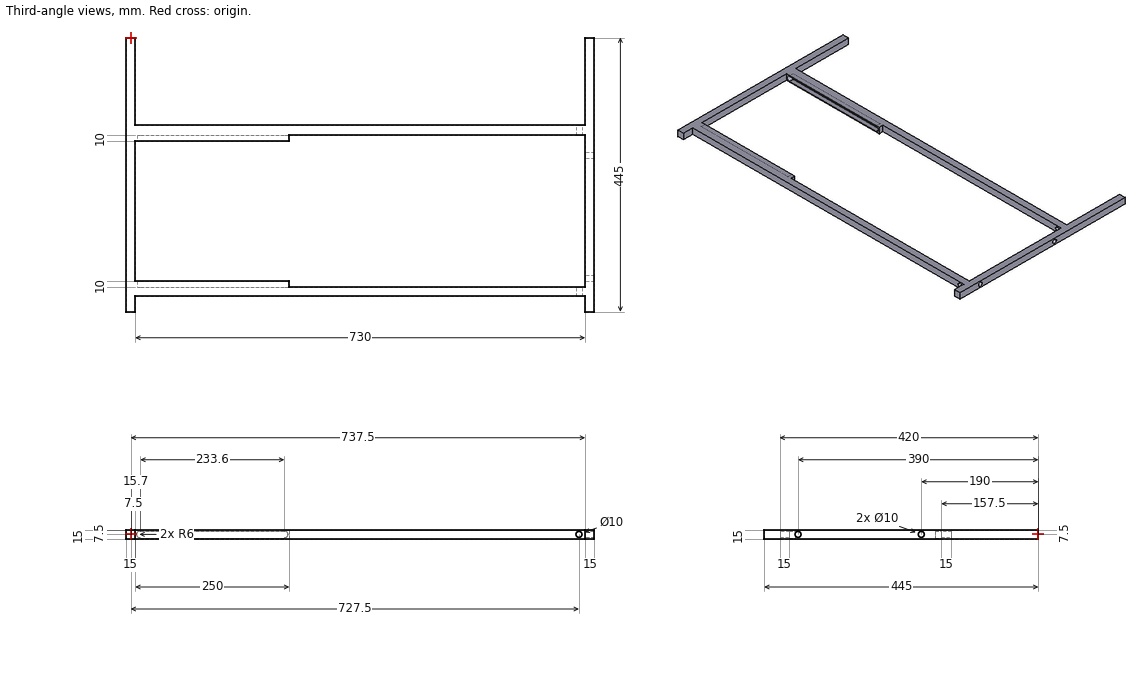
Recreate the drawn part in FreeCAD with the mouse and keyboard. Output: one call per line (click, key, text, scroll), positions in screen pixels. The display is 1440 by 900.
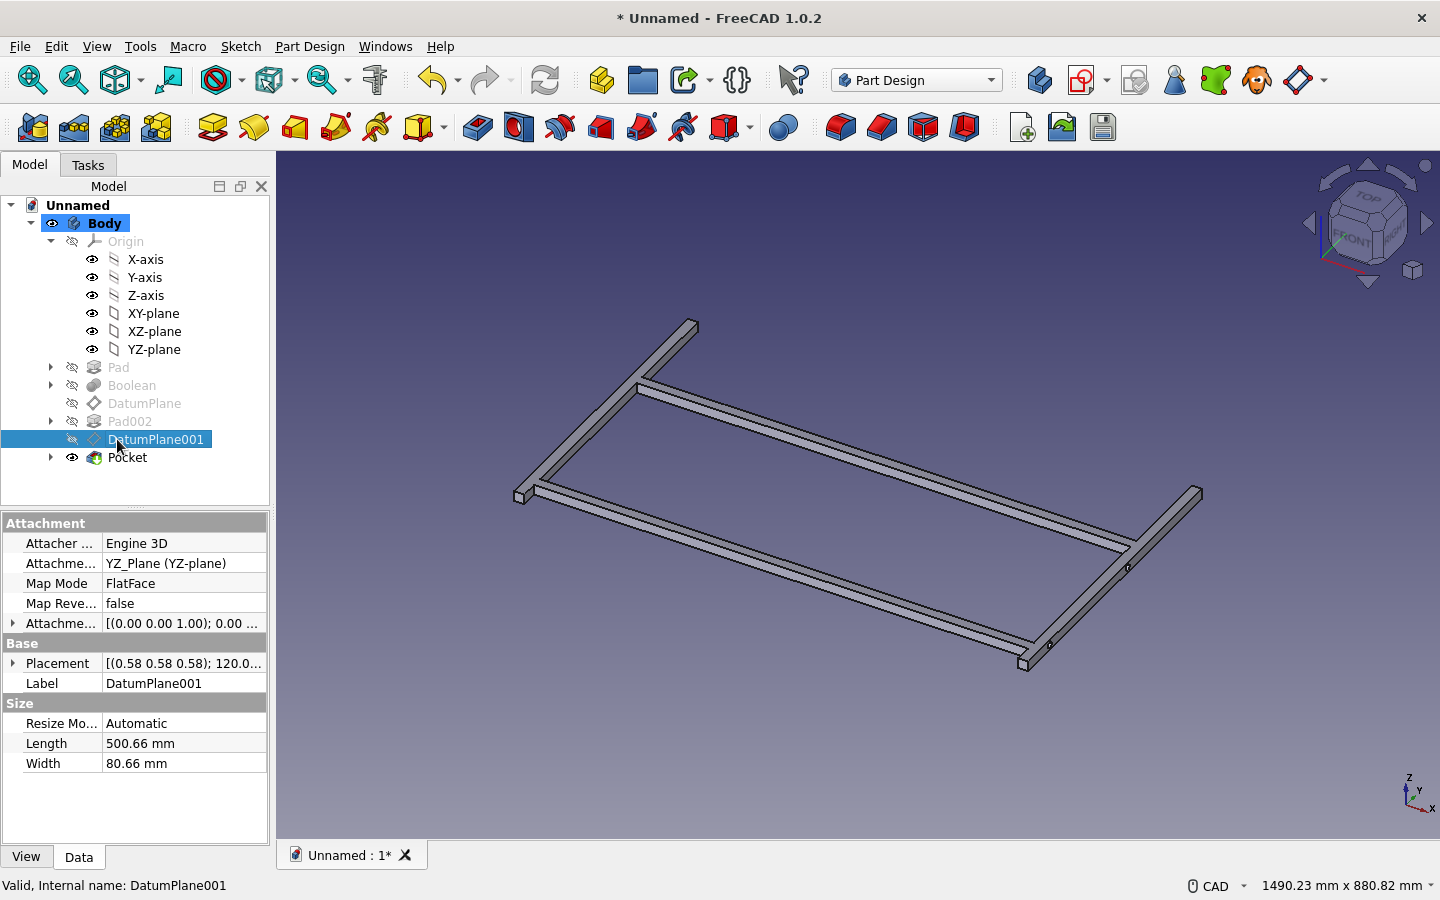
click(137, 331)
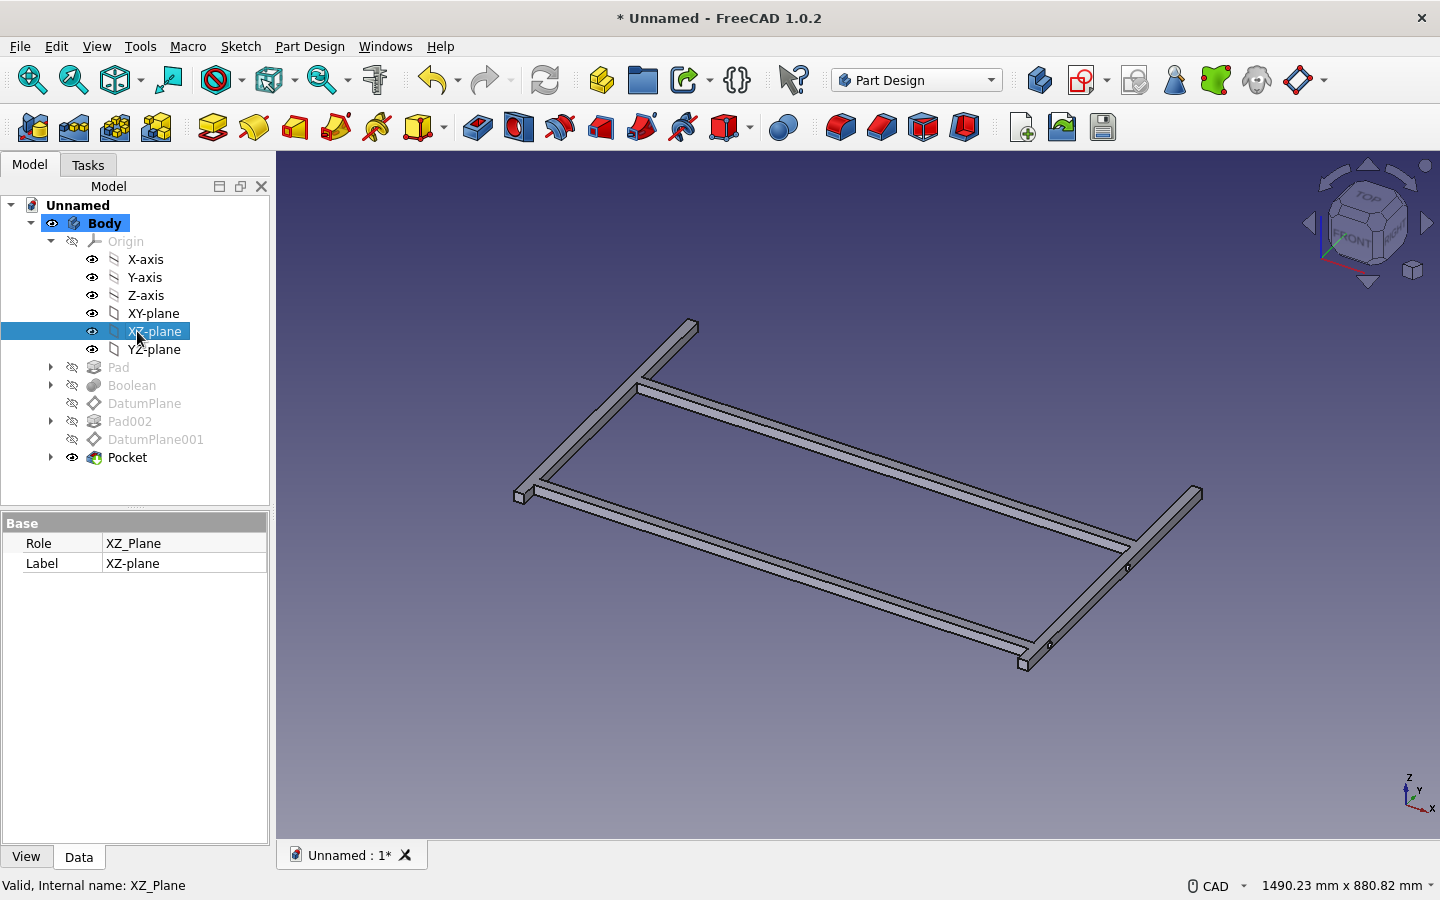
click(1298, 80)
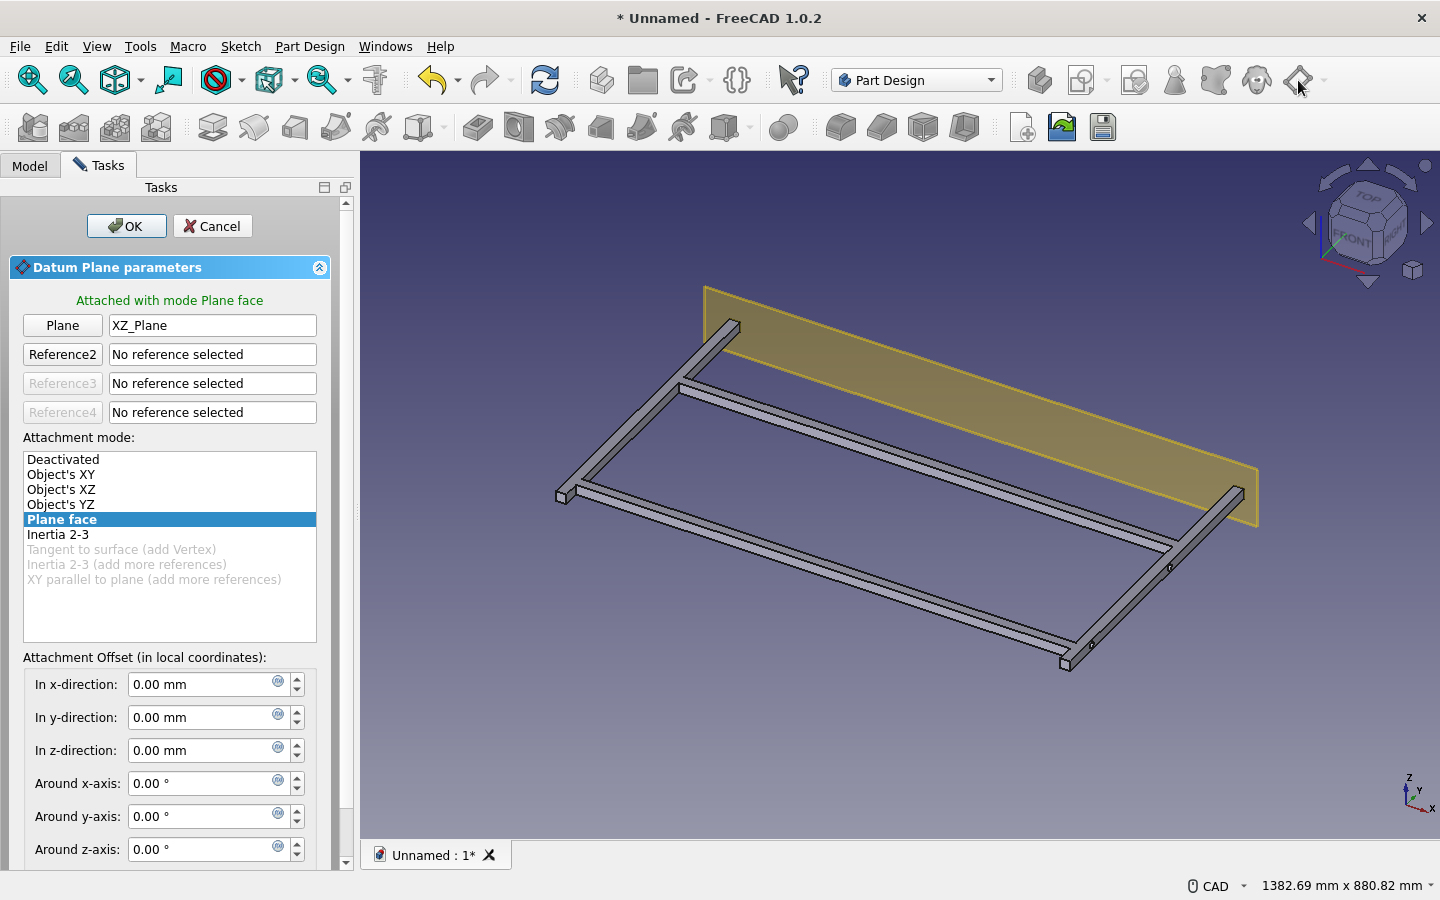
triple_click(210, 750)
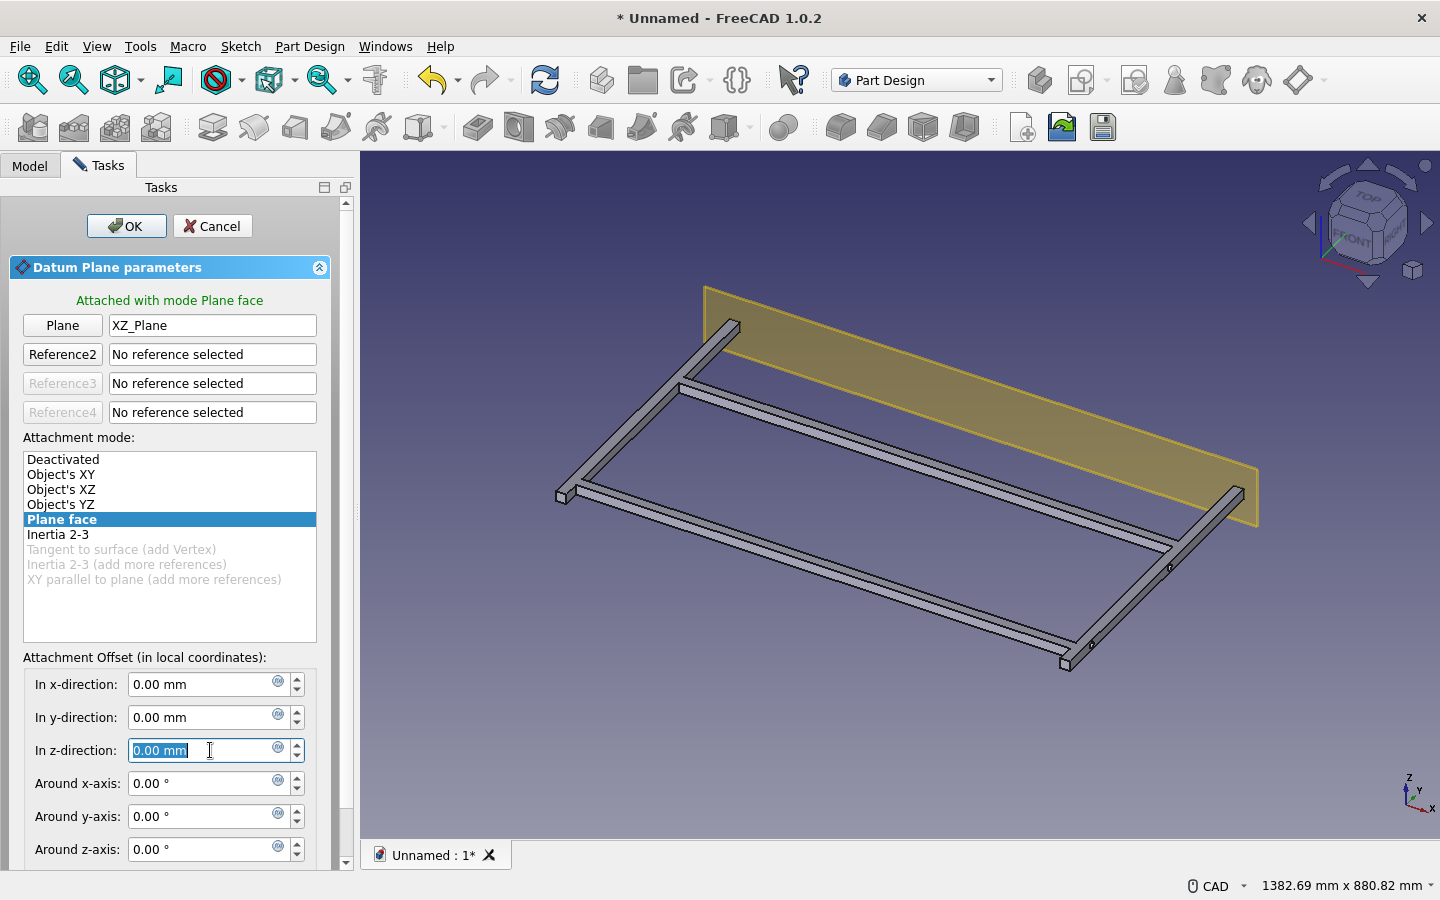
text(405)
key(Tab)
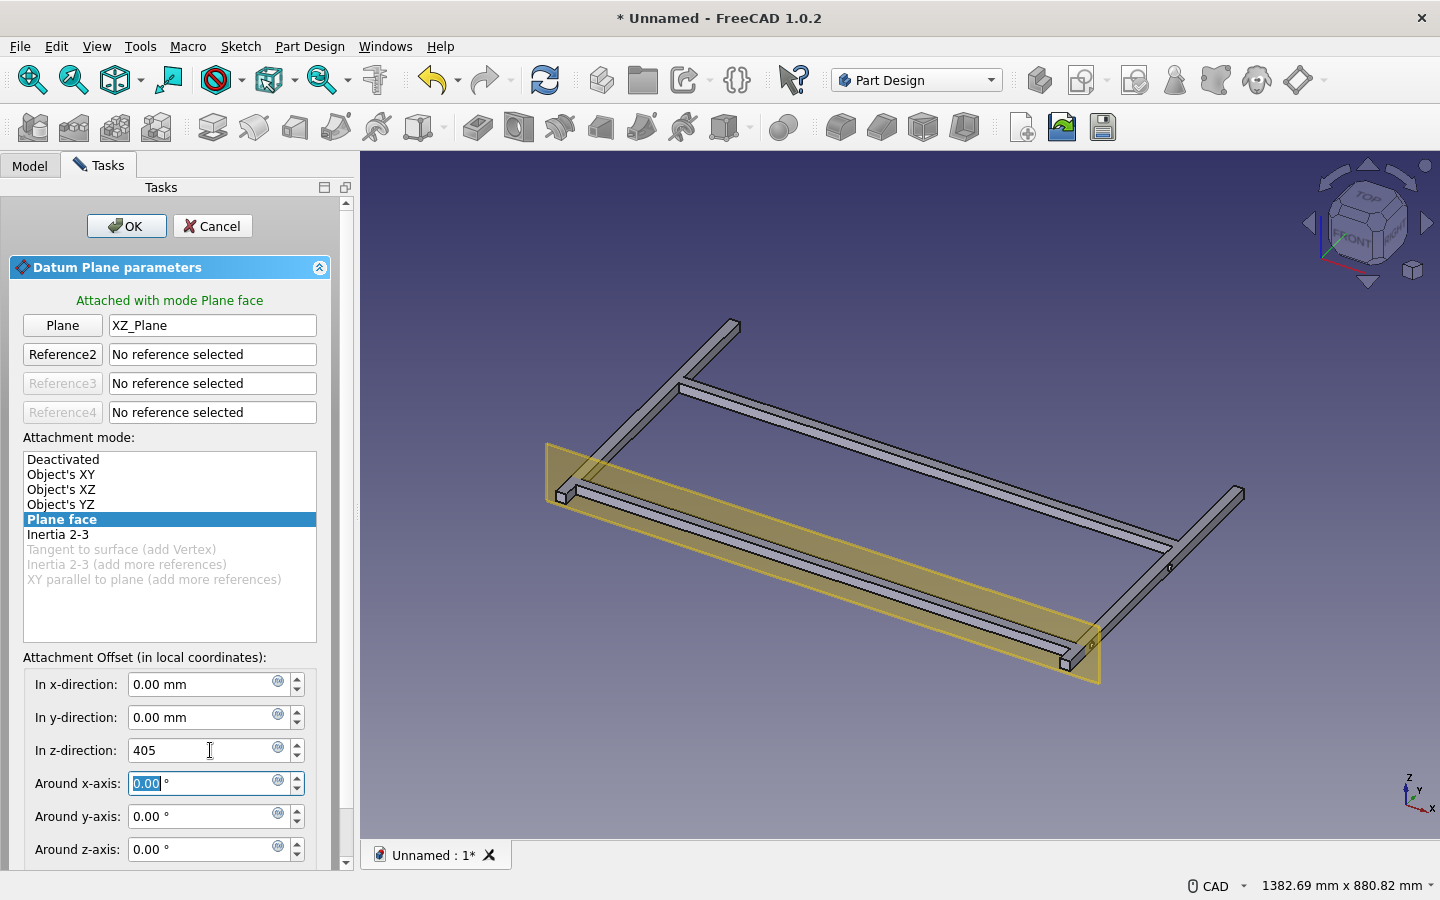
click(127, 226)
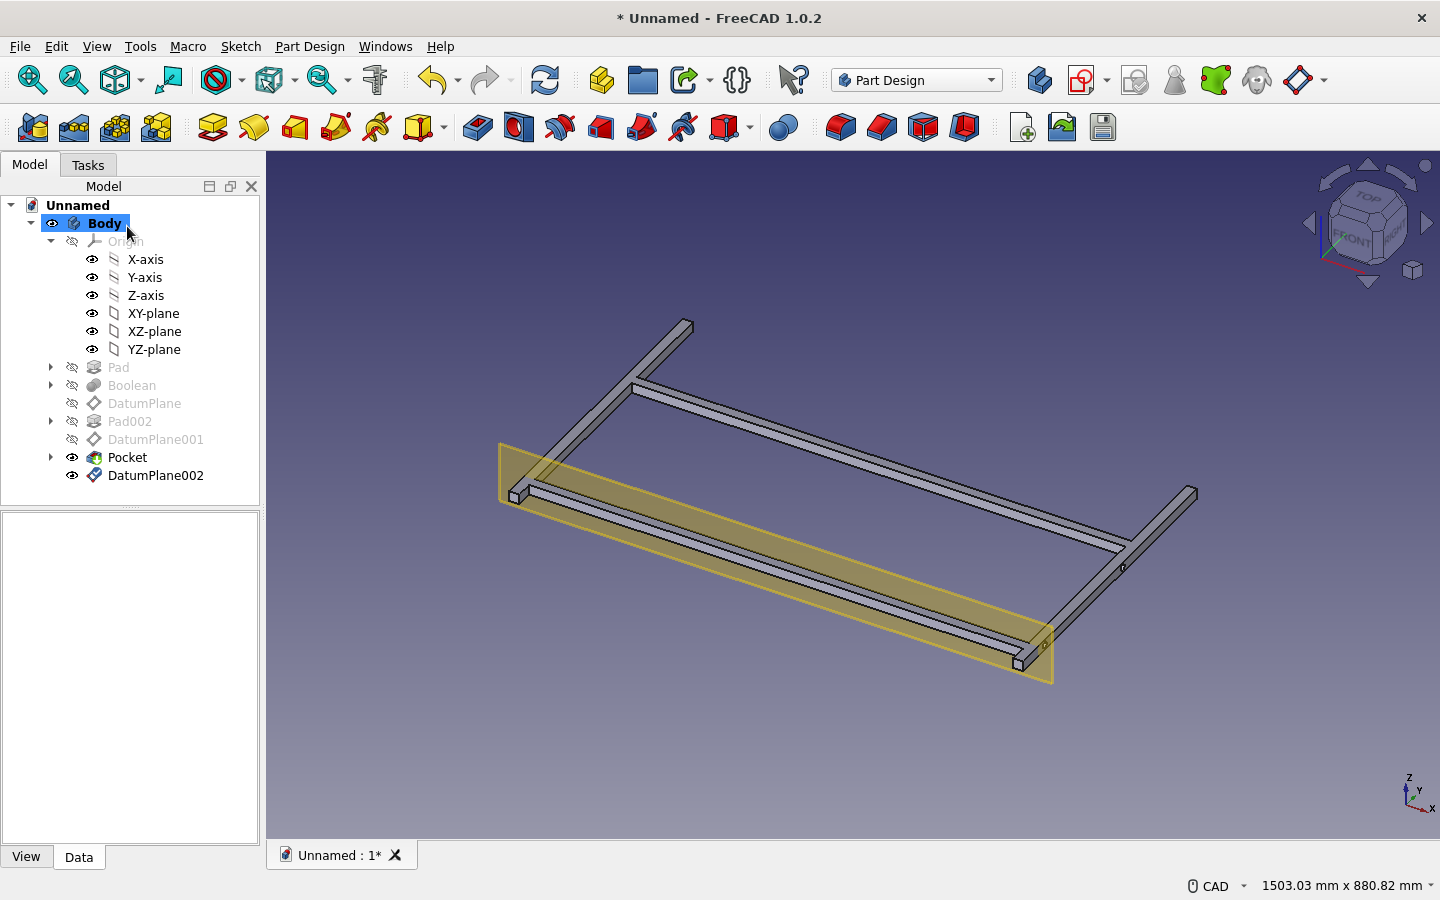
click(117, 475)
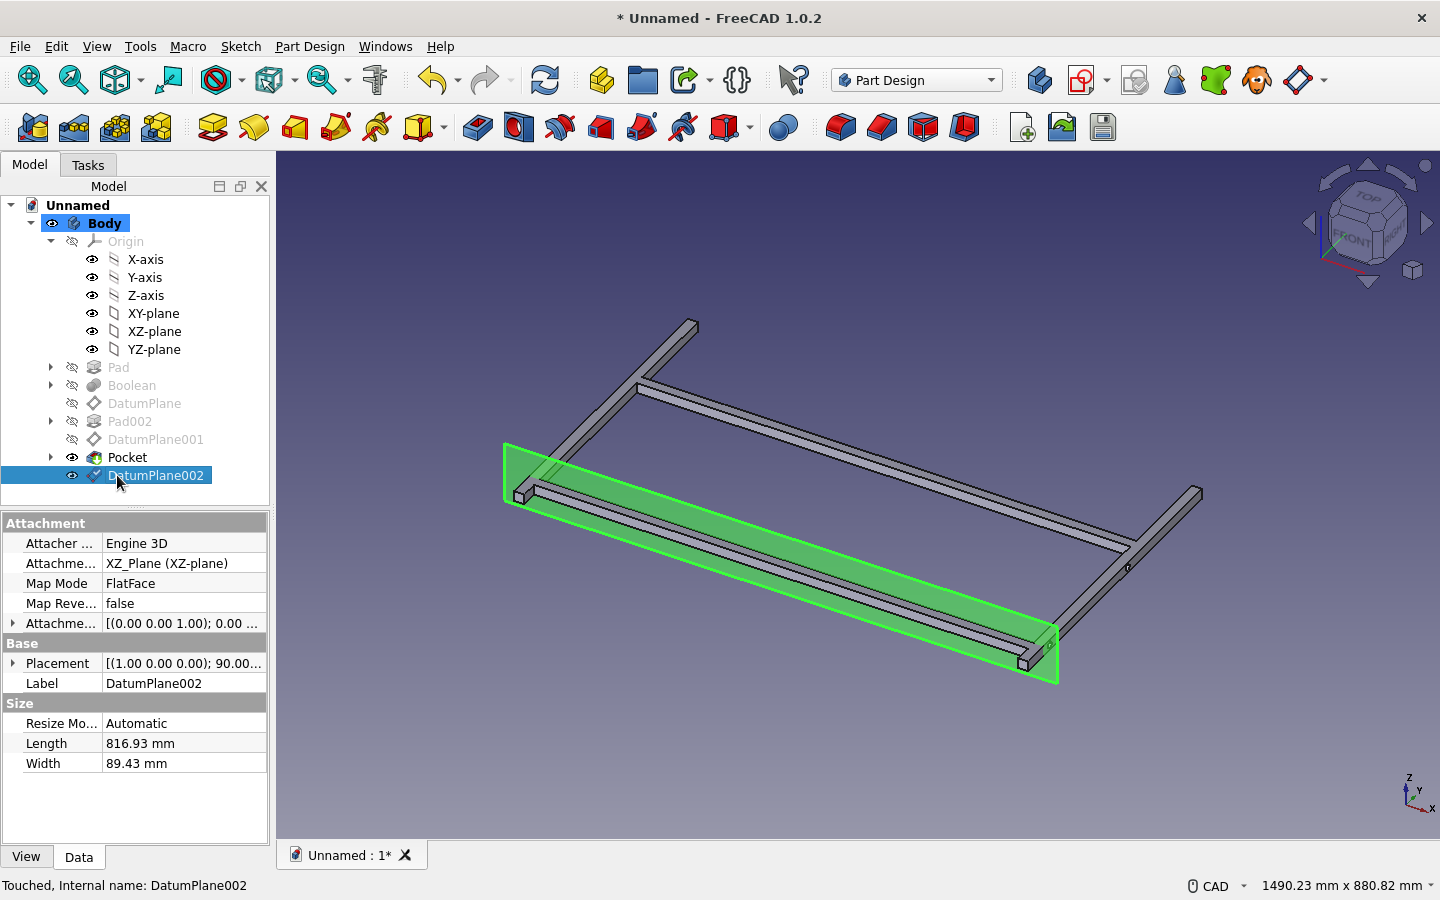
click(1080, 80)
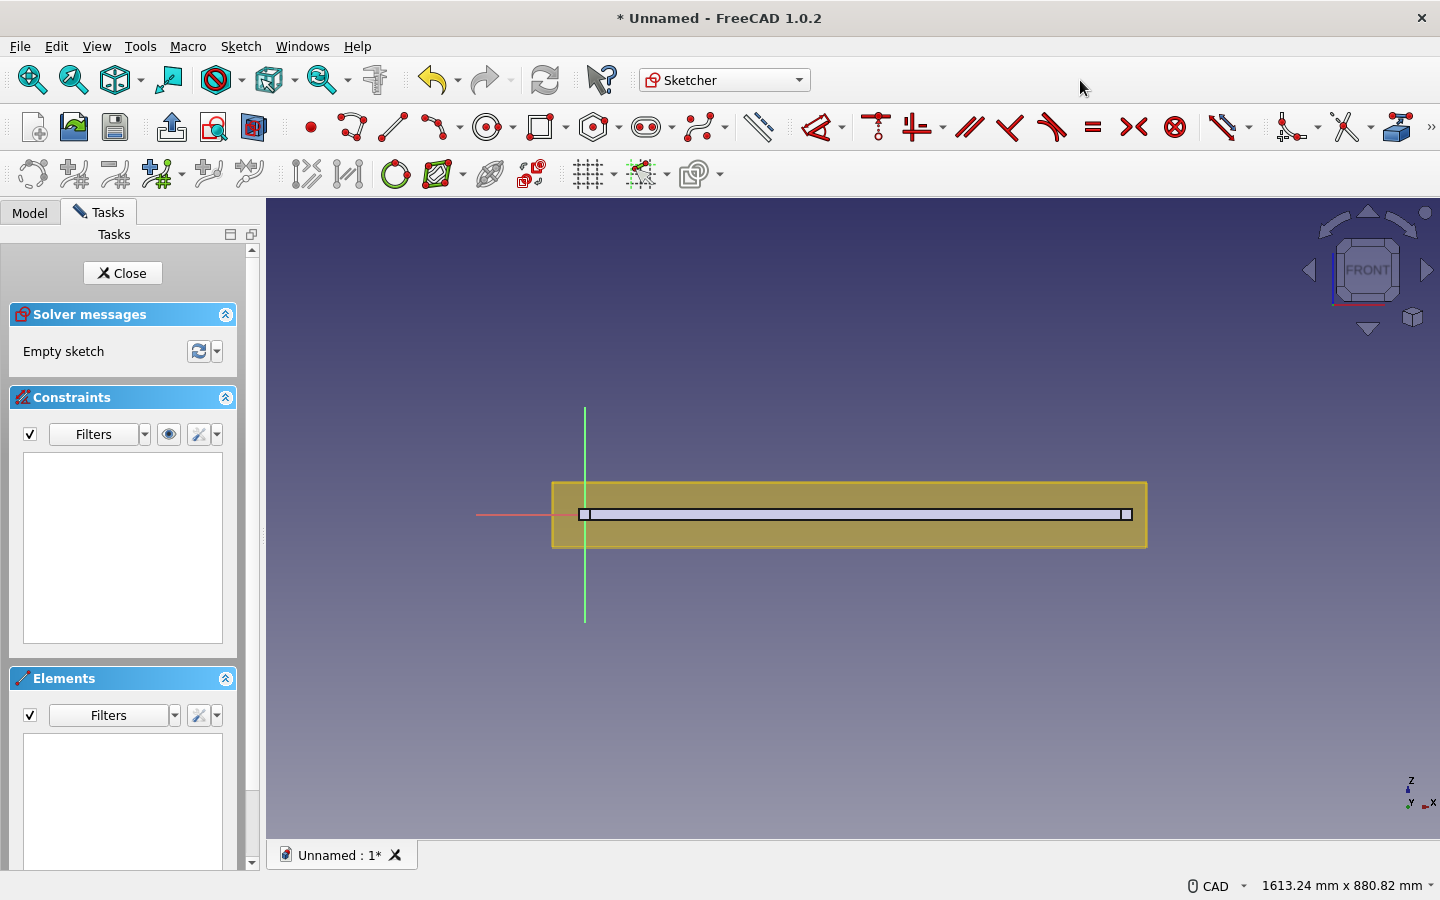
click(254, 128)